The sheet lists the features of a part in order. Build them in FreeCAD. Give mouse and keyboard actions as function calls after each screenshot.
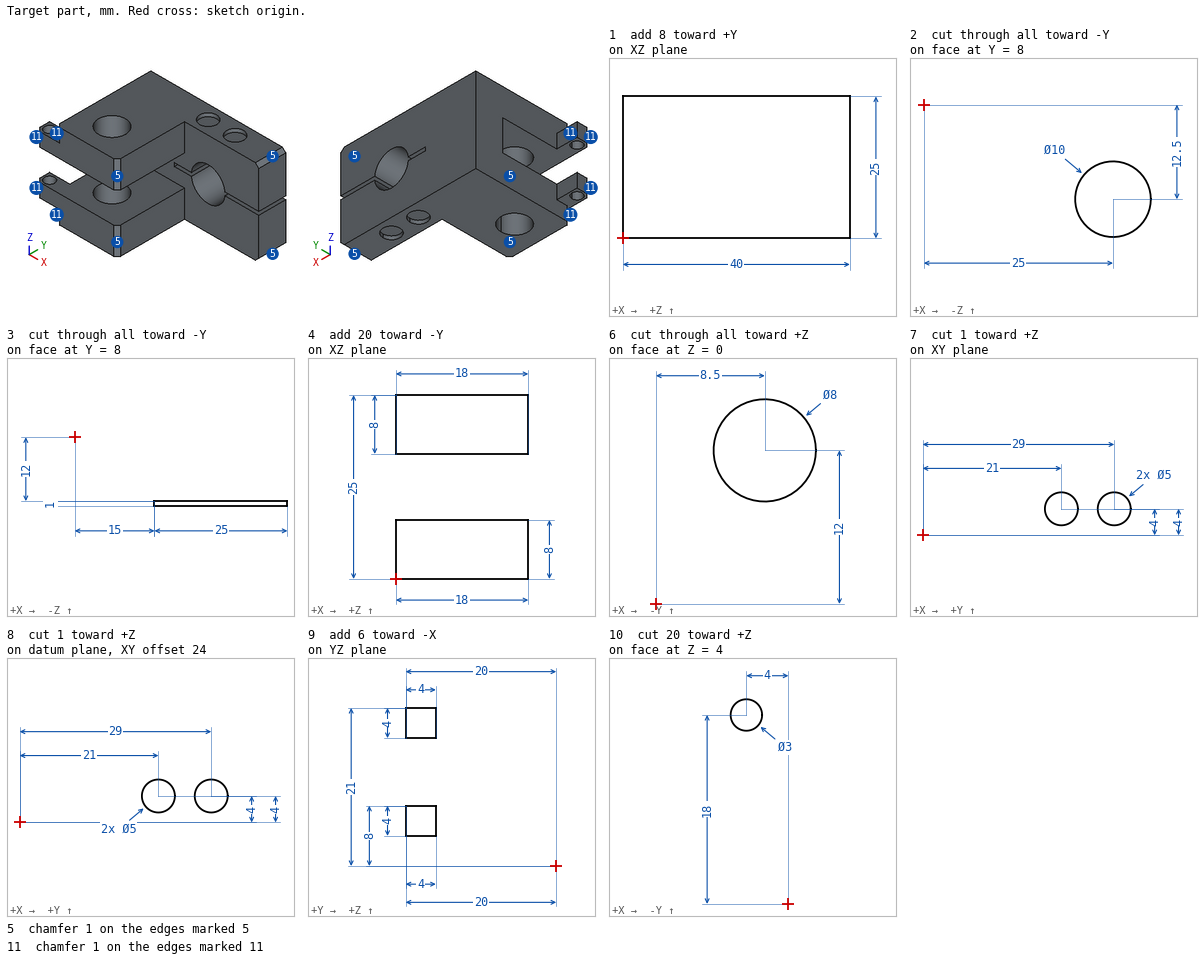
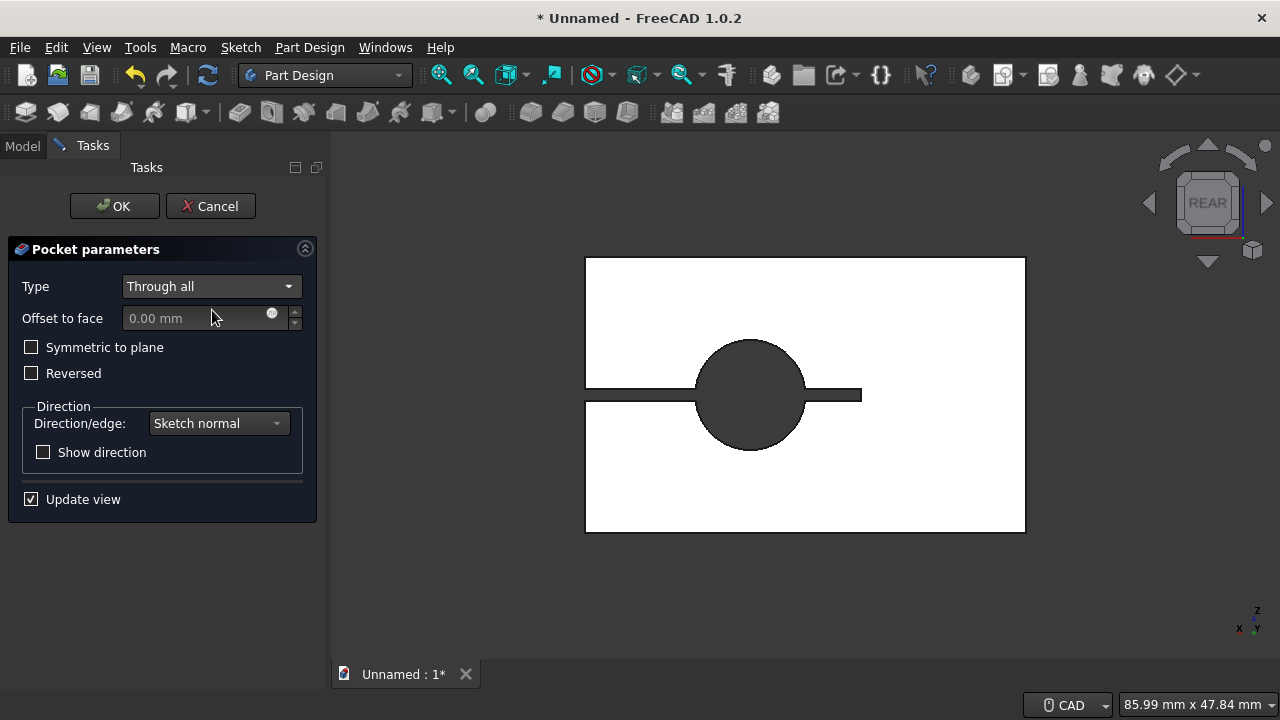
click(115, 206)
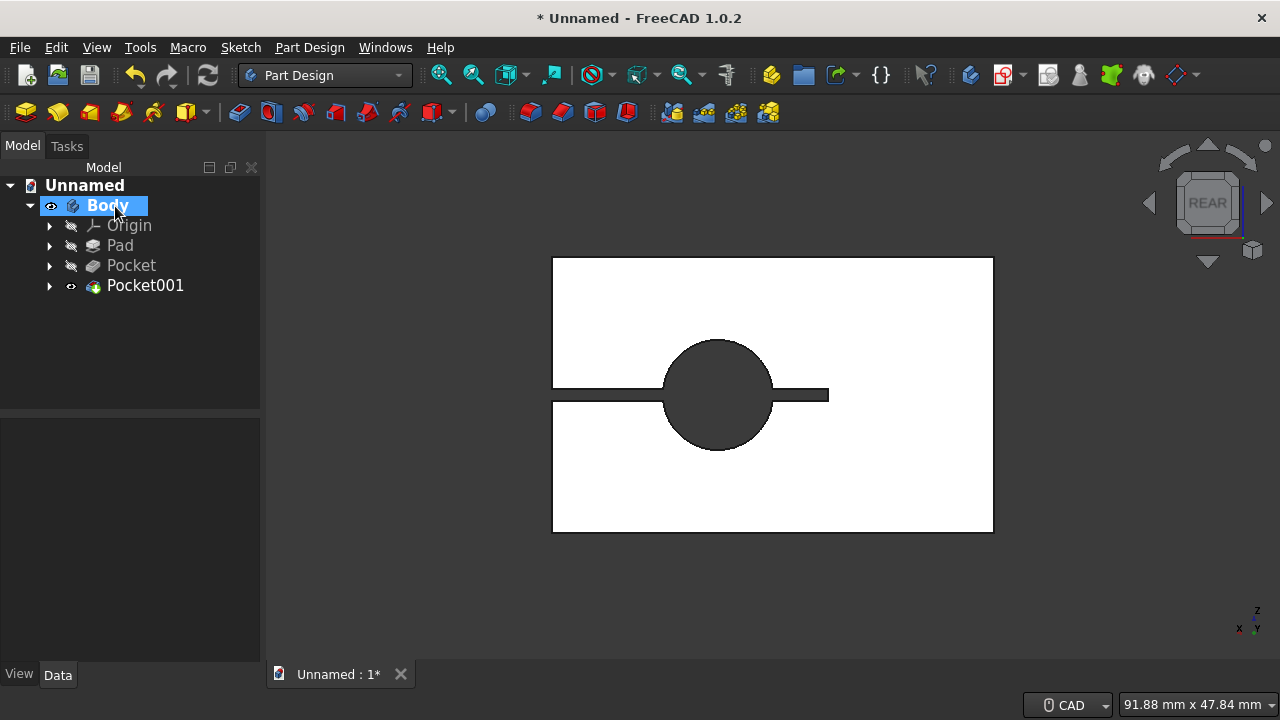
click(1004, 76)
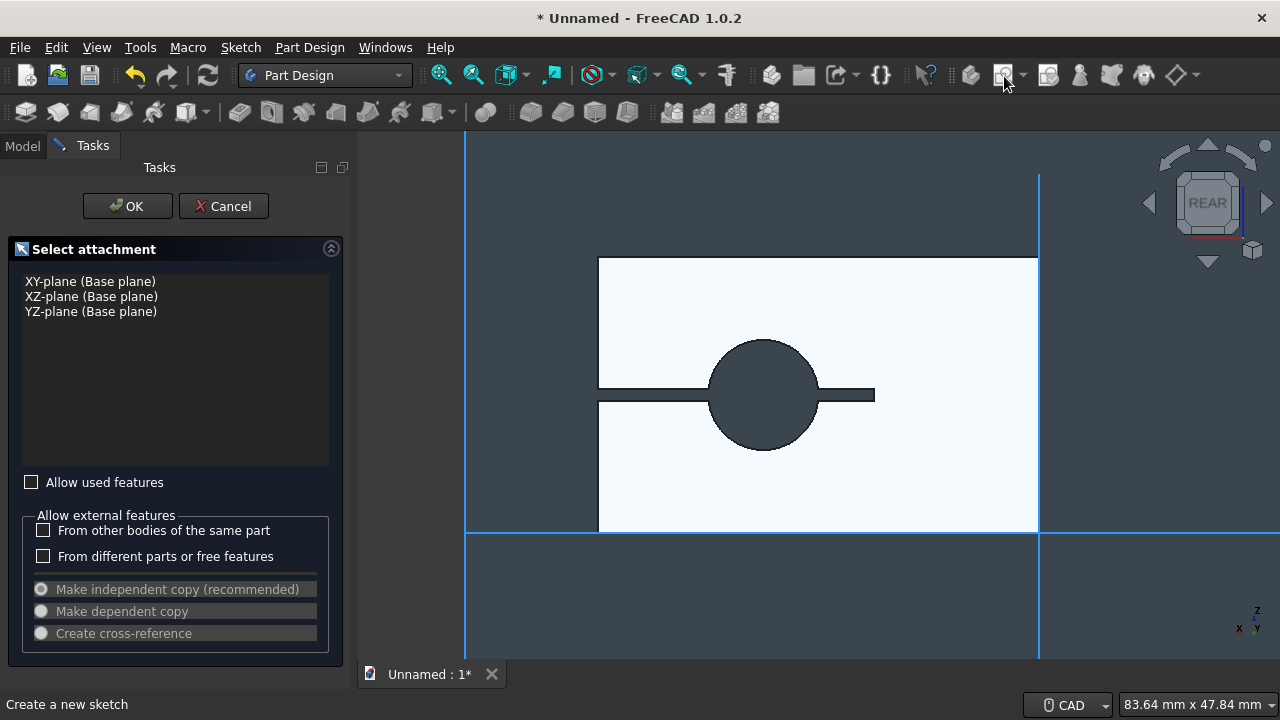
click(82, 296)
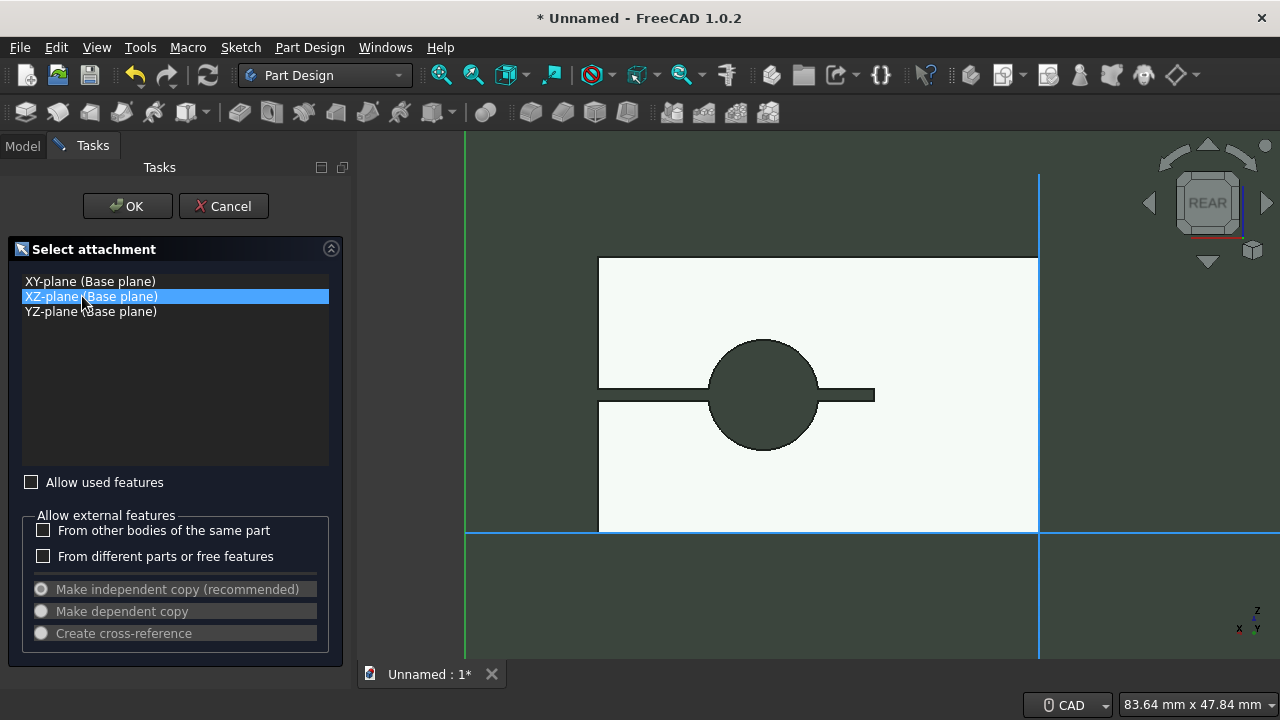
click(128, 206)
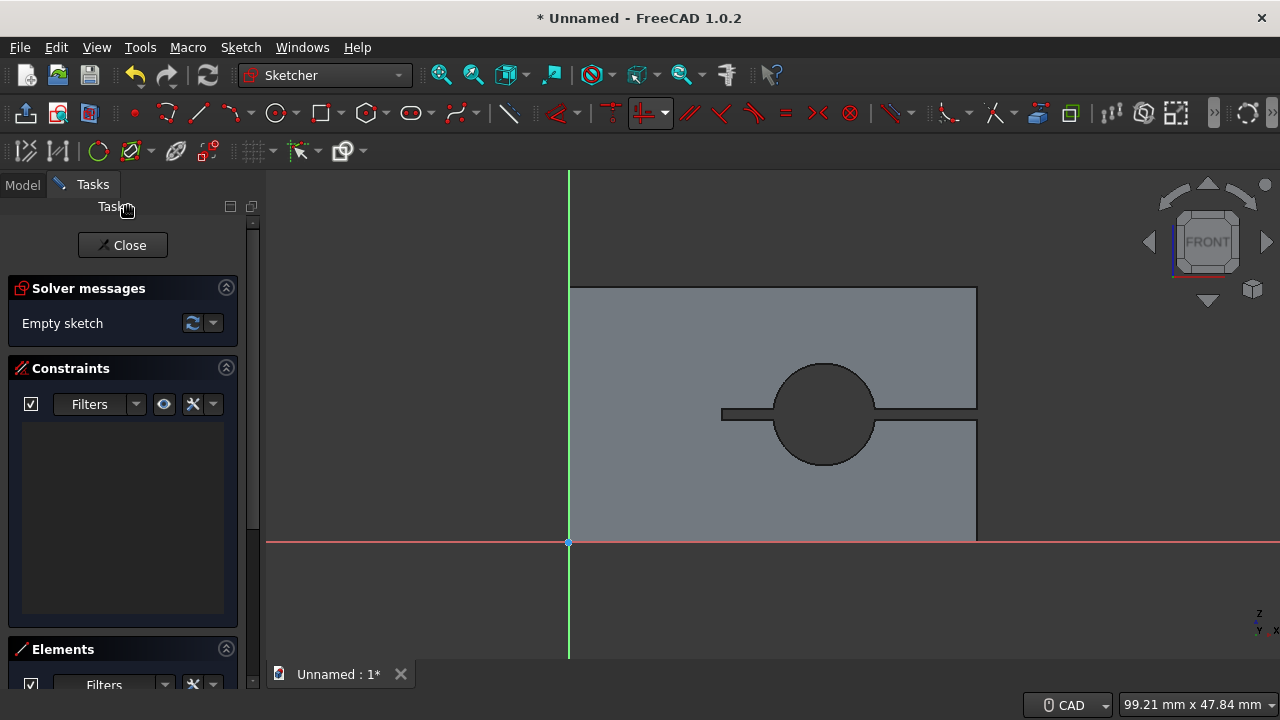
click(322, 114)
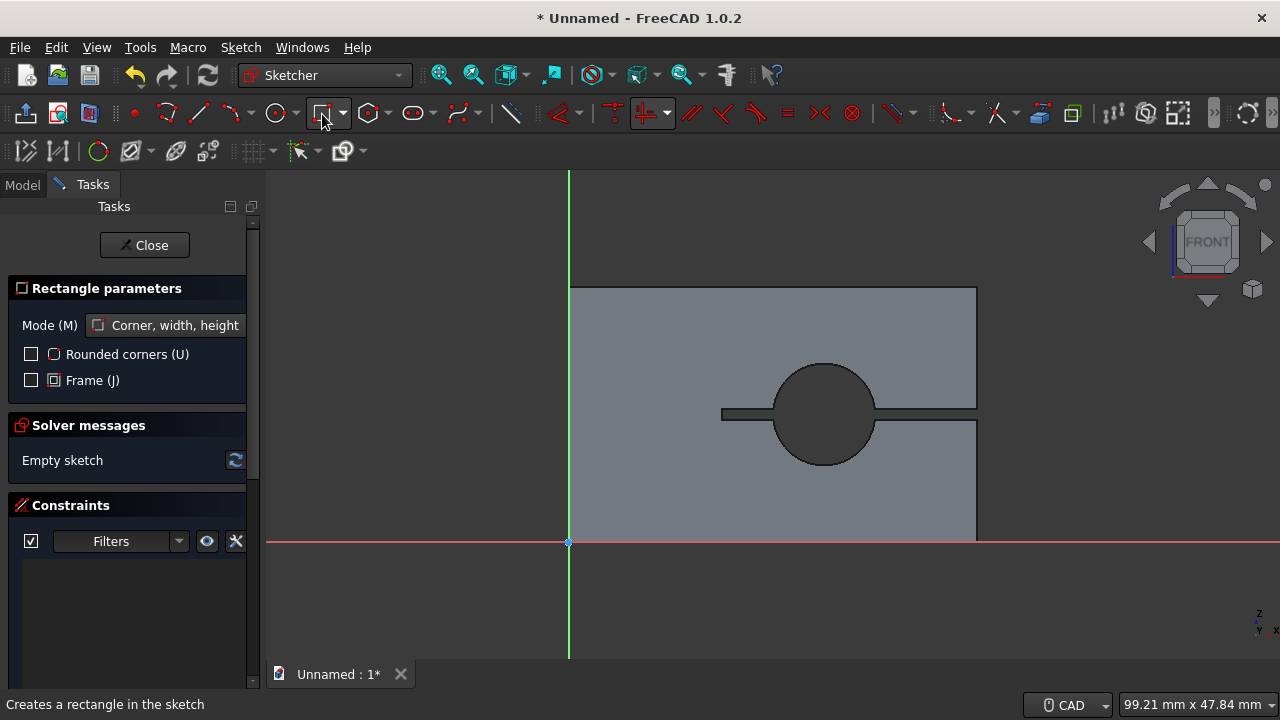
click(569, 542)
click(753, 460)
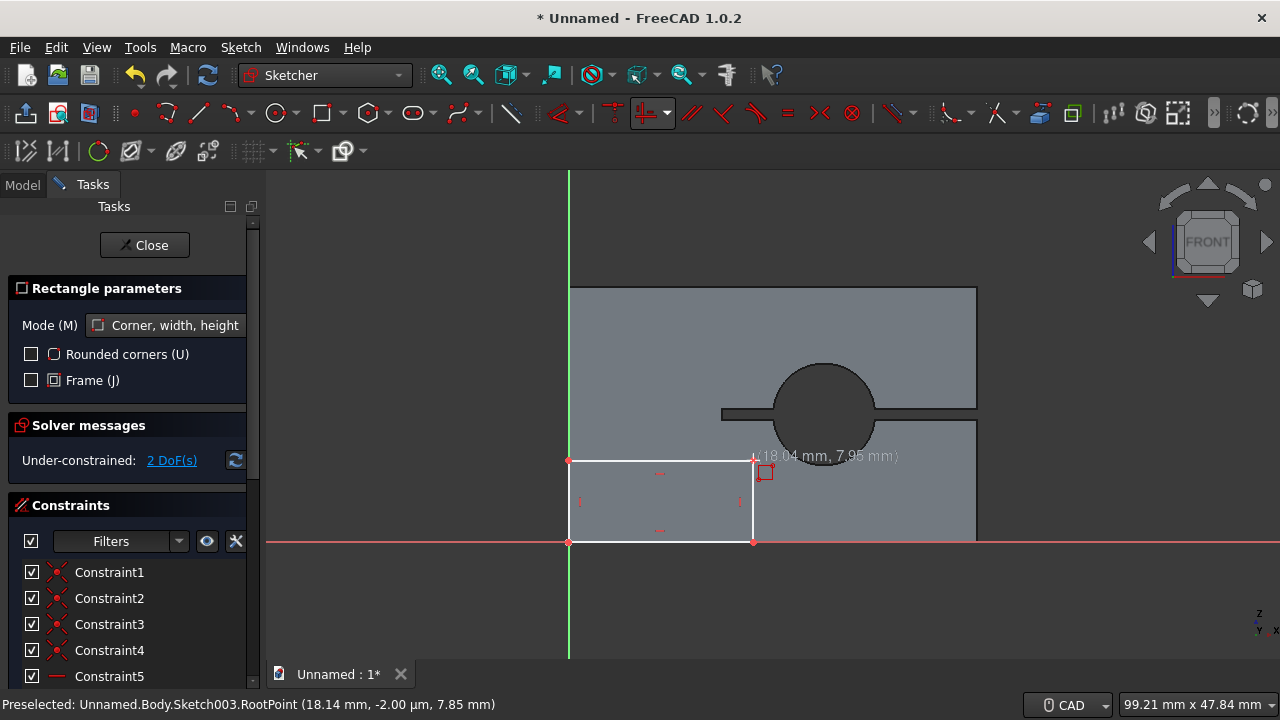
click(569, 287)
click(753, 369)
key(Escape)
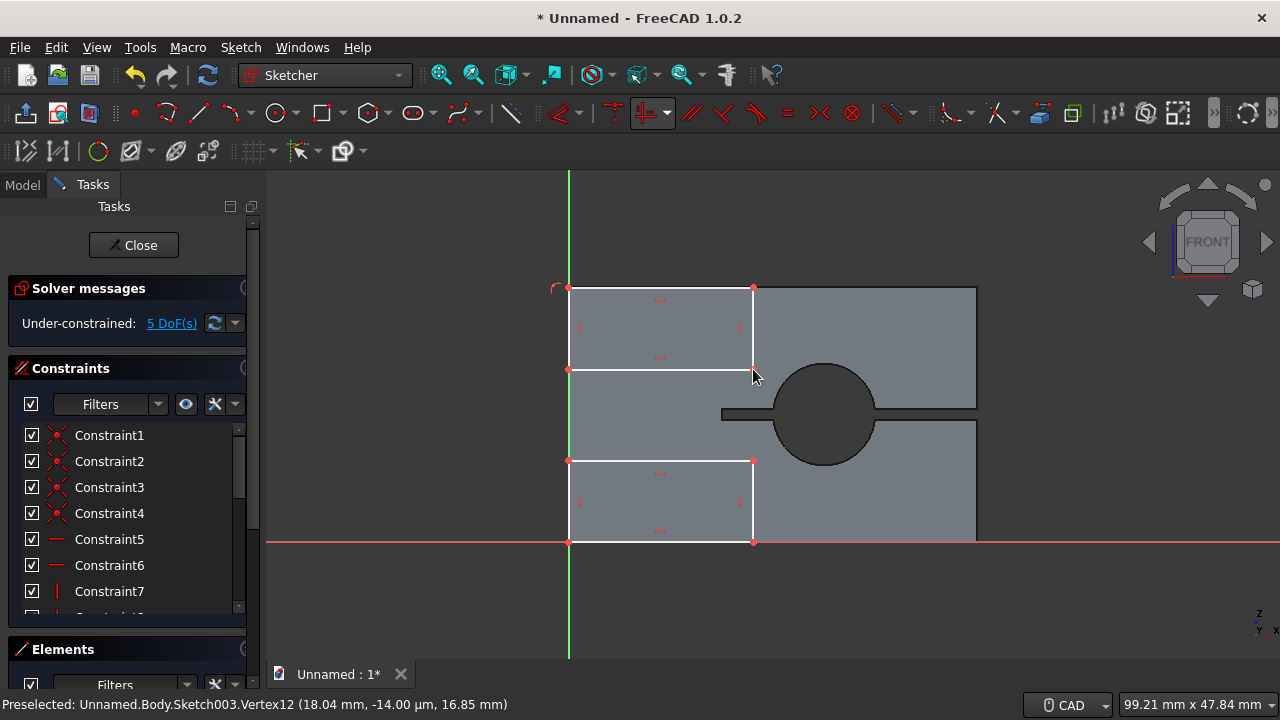
click(558, 114)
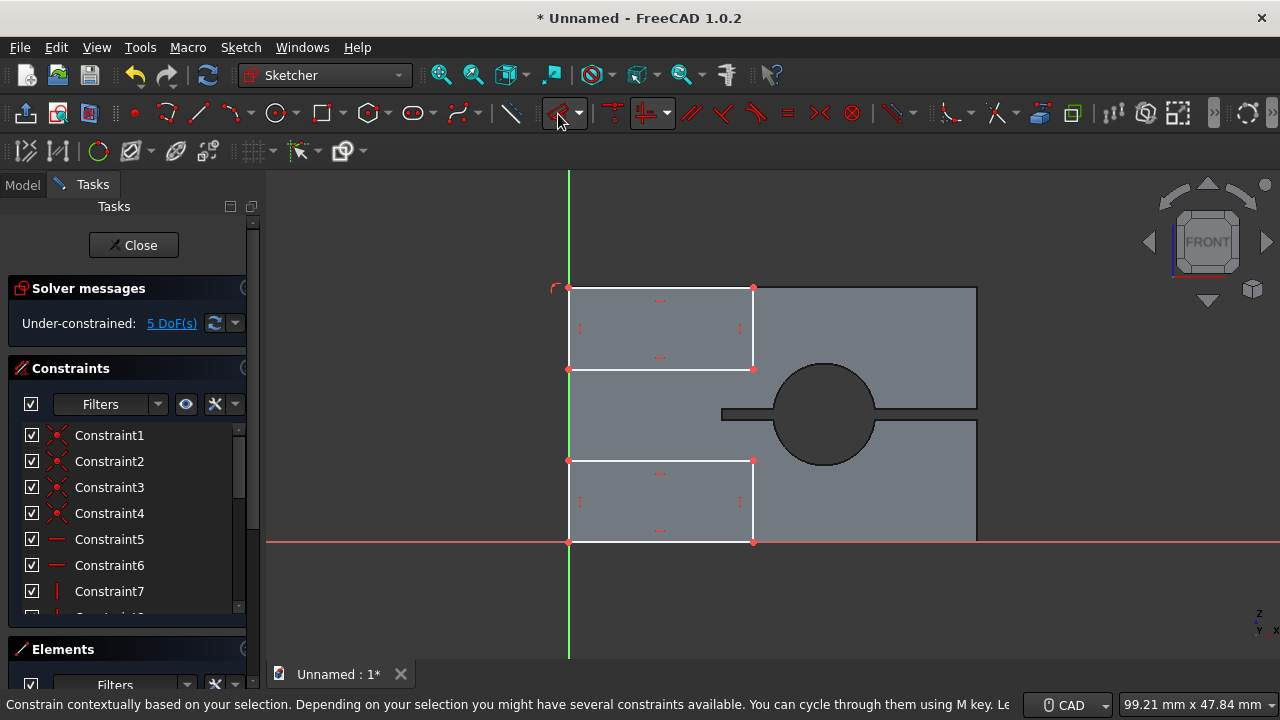
click(753, 518)
click(787, 502)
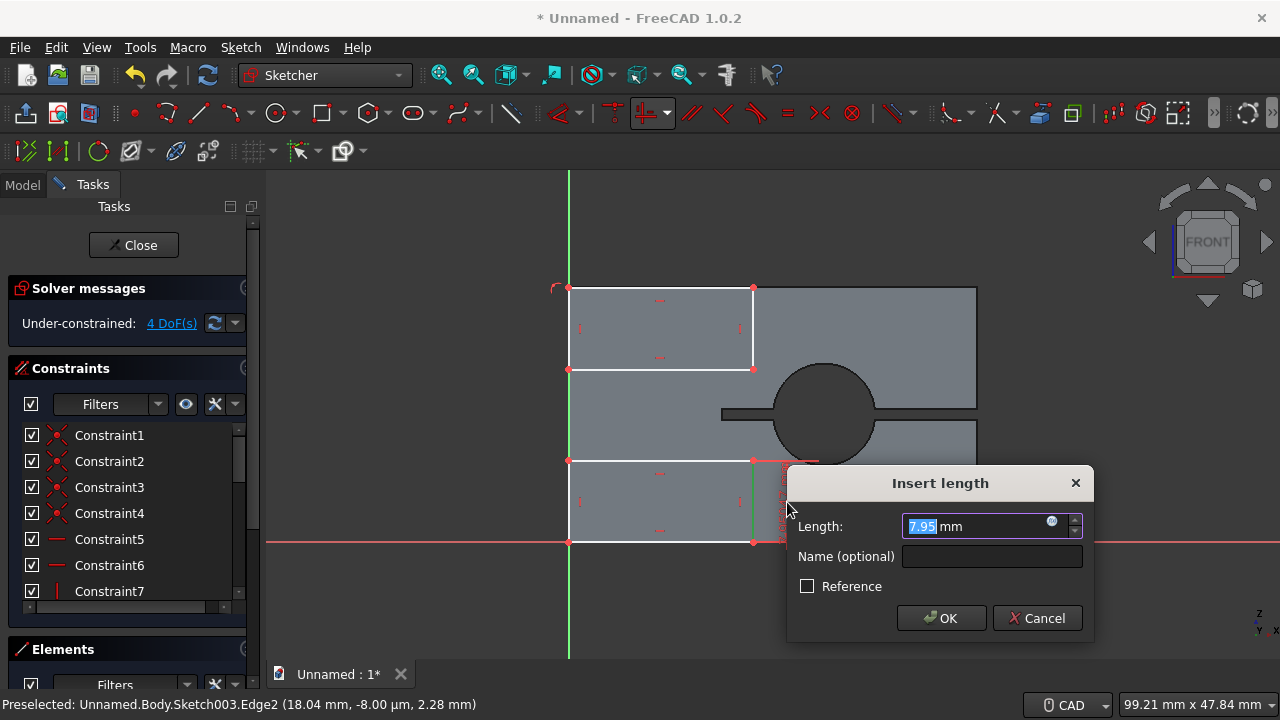
text(8)
key(Return)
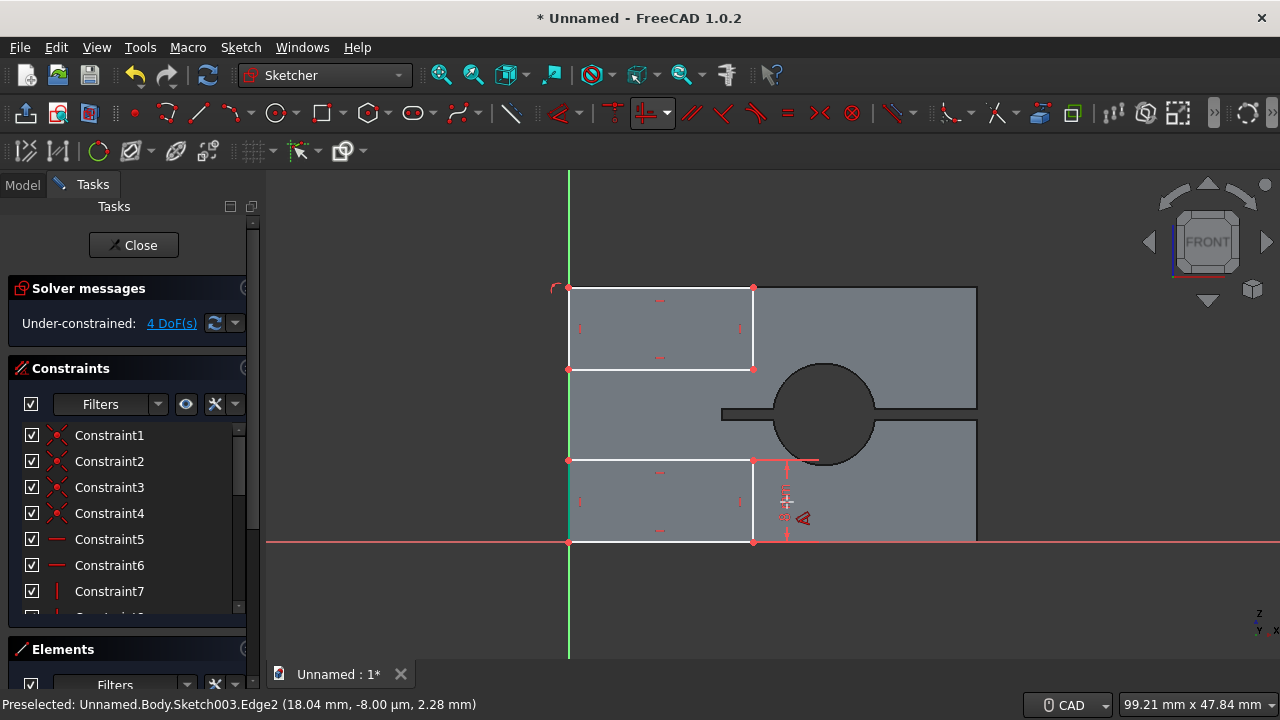
click(569, 313)
click(535, 329)